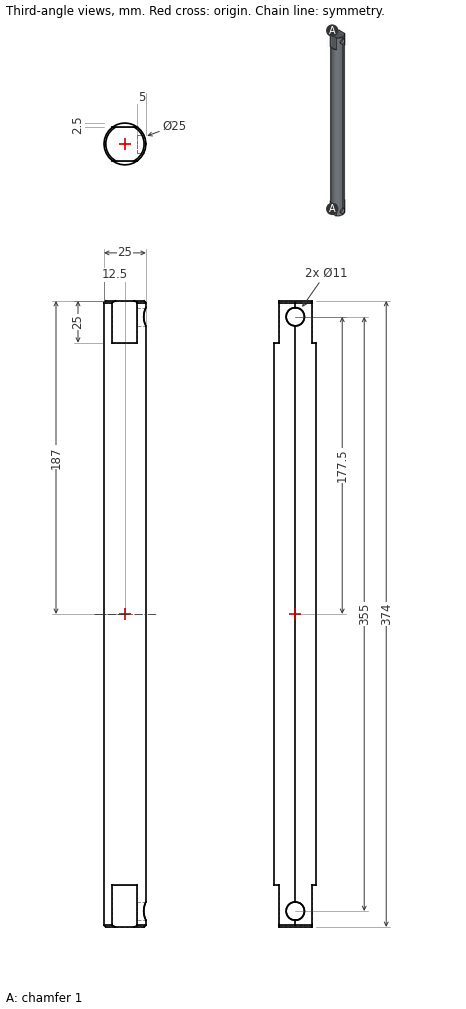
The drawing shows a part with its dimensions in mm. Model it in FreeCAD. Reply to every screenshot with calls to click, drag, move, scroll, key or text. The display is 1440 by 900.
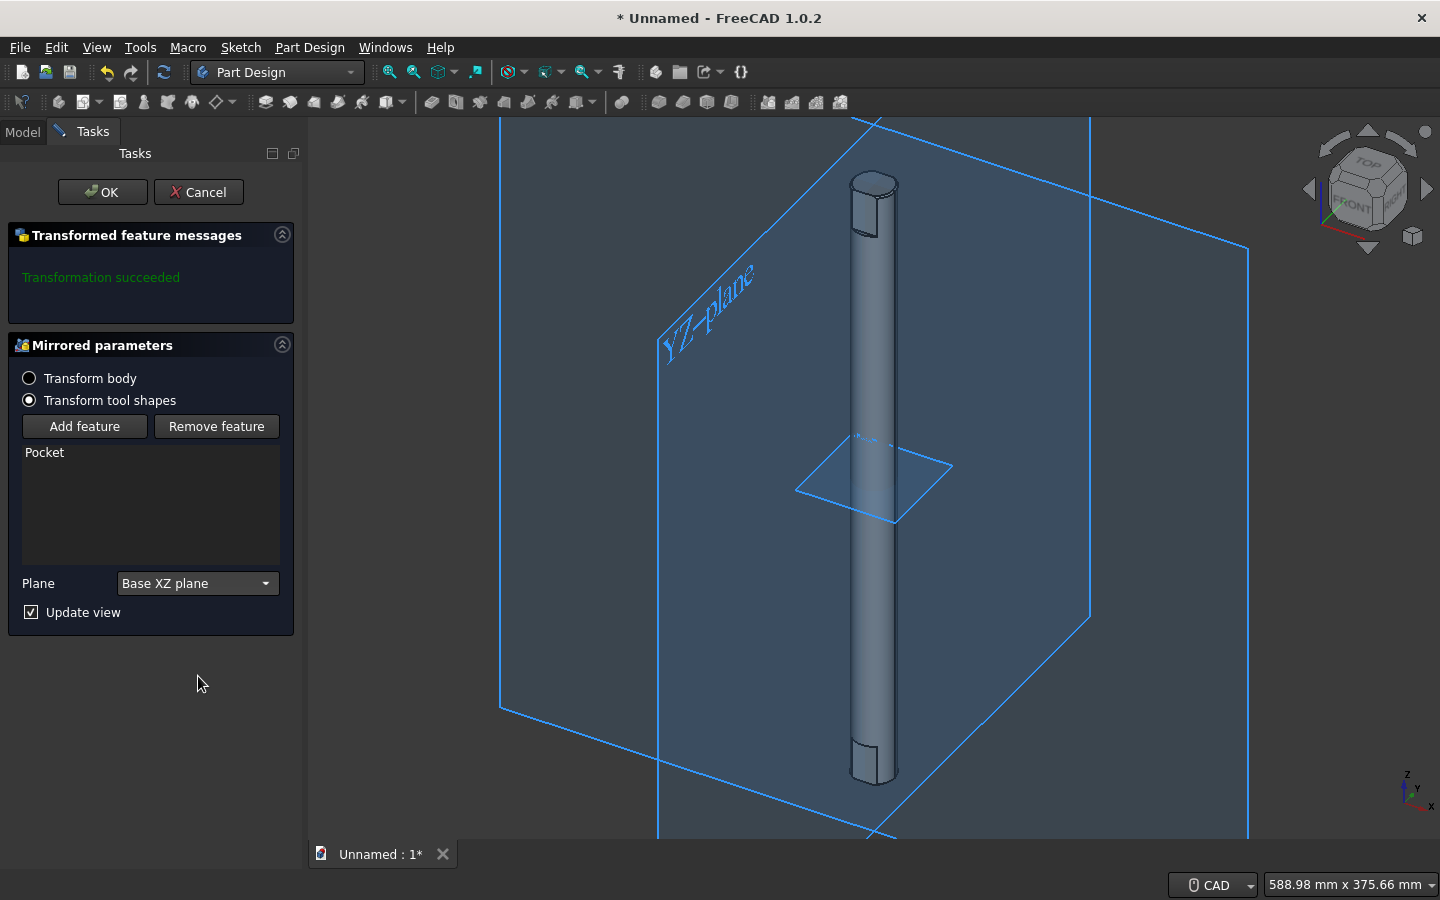
click(103, 192)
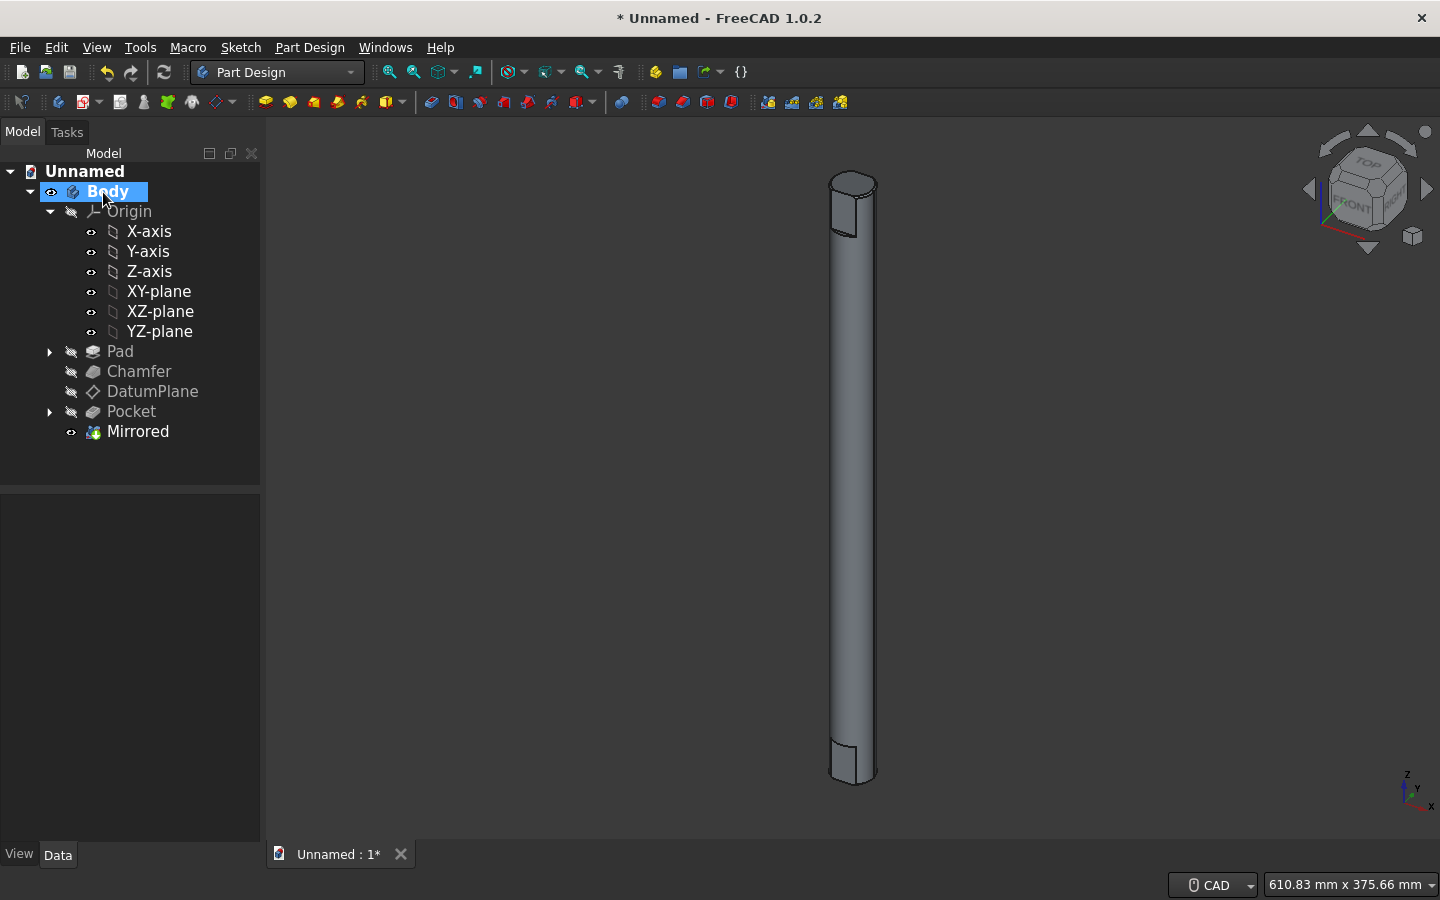
click(136, 332)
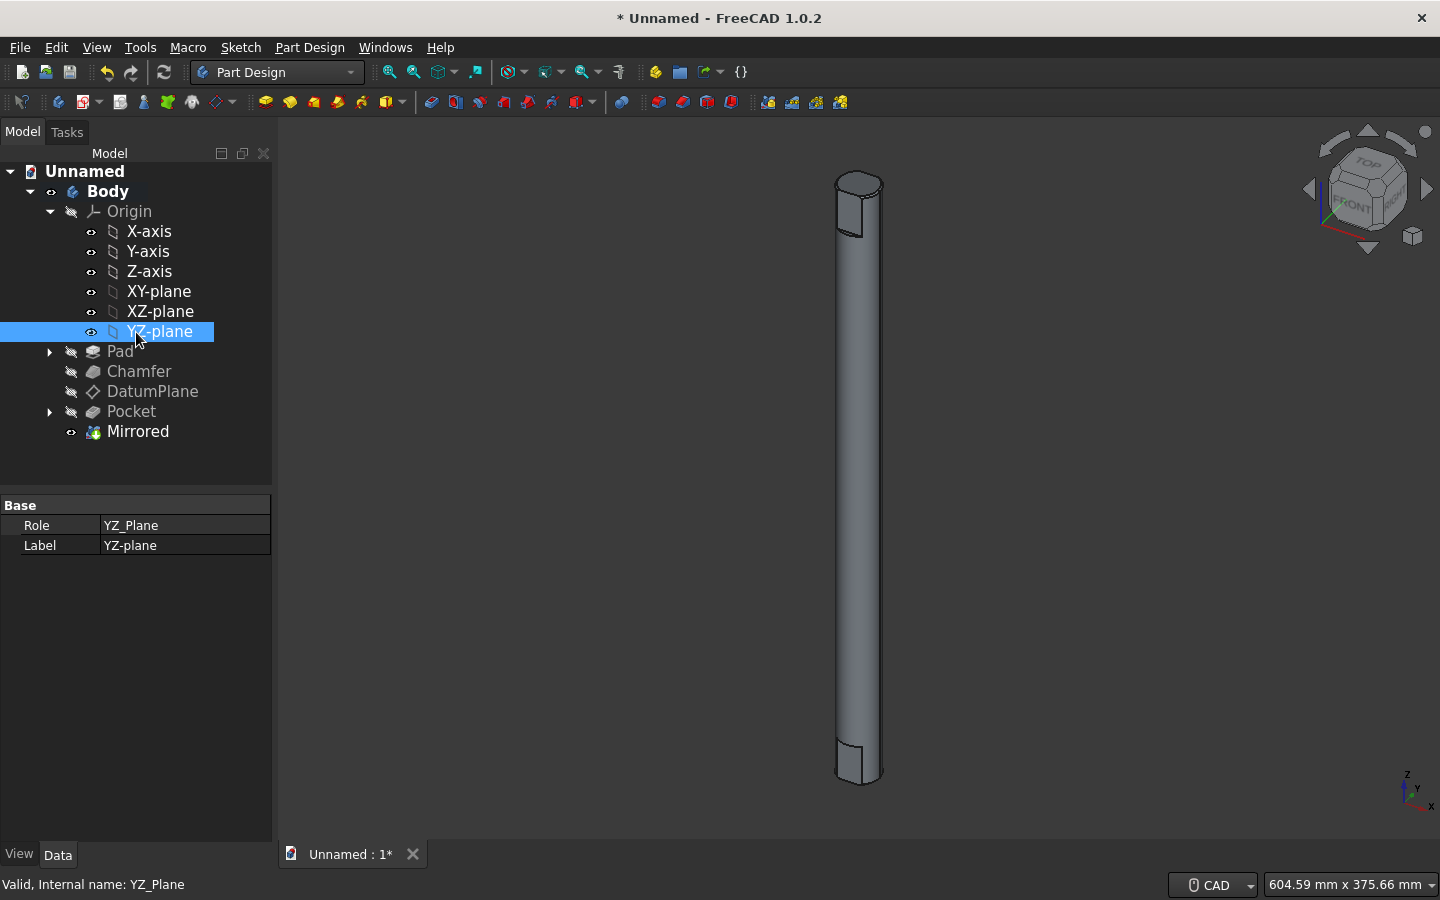
click(216, 102)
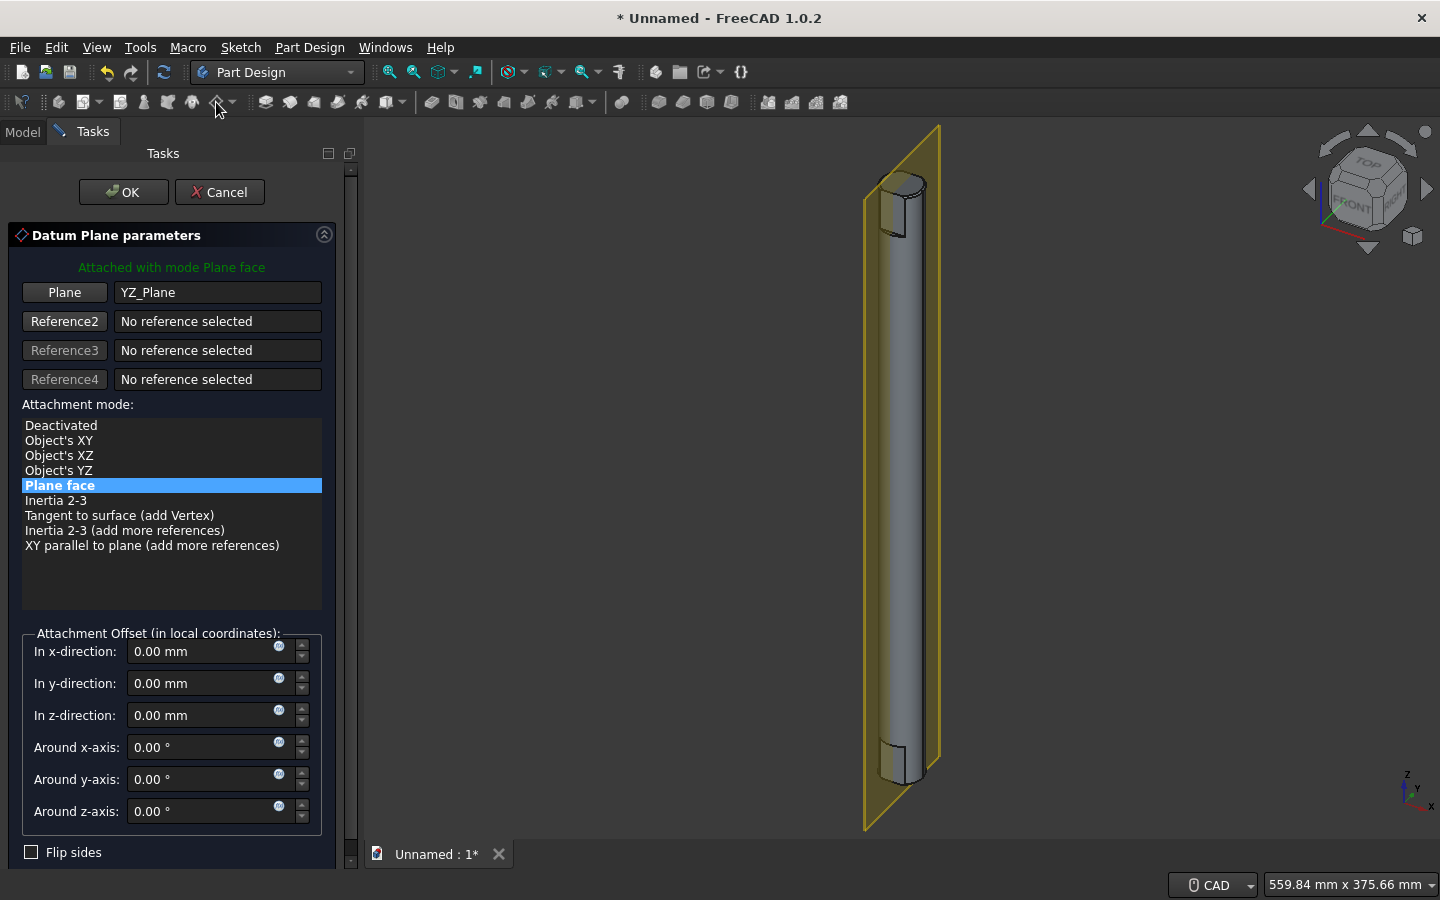
triple_click(210, 715)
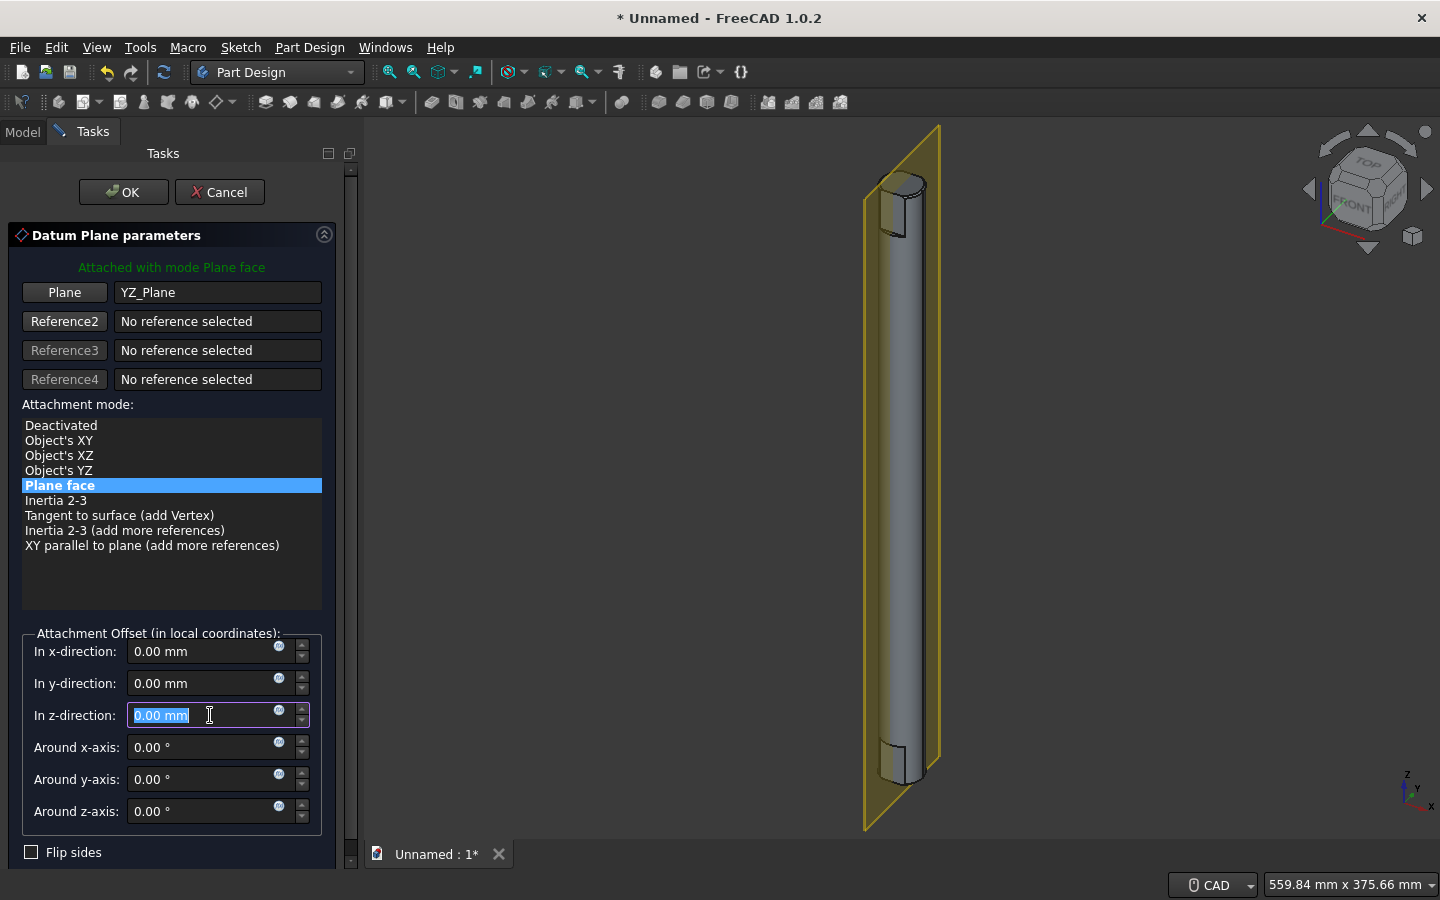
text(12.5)
key(Tab)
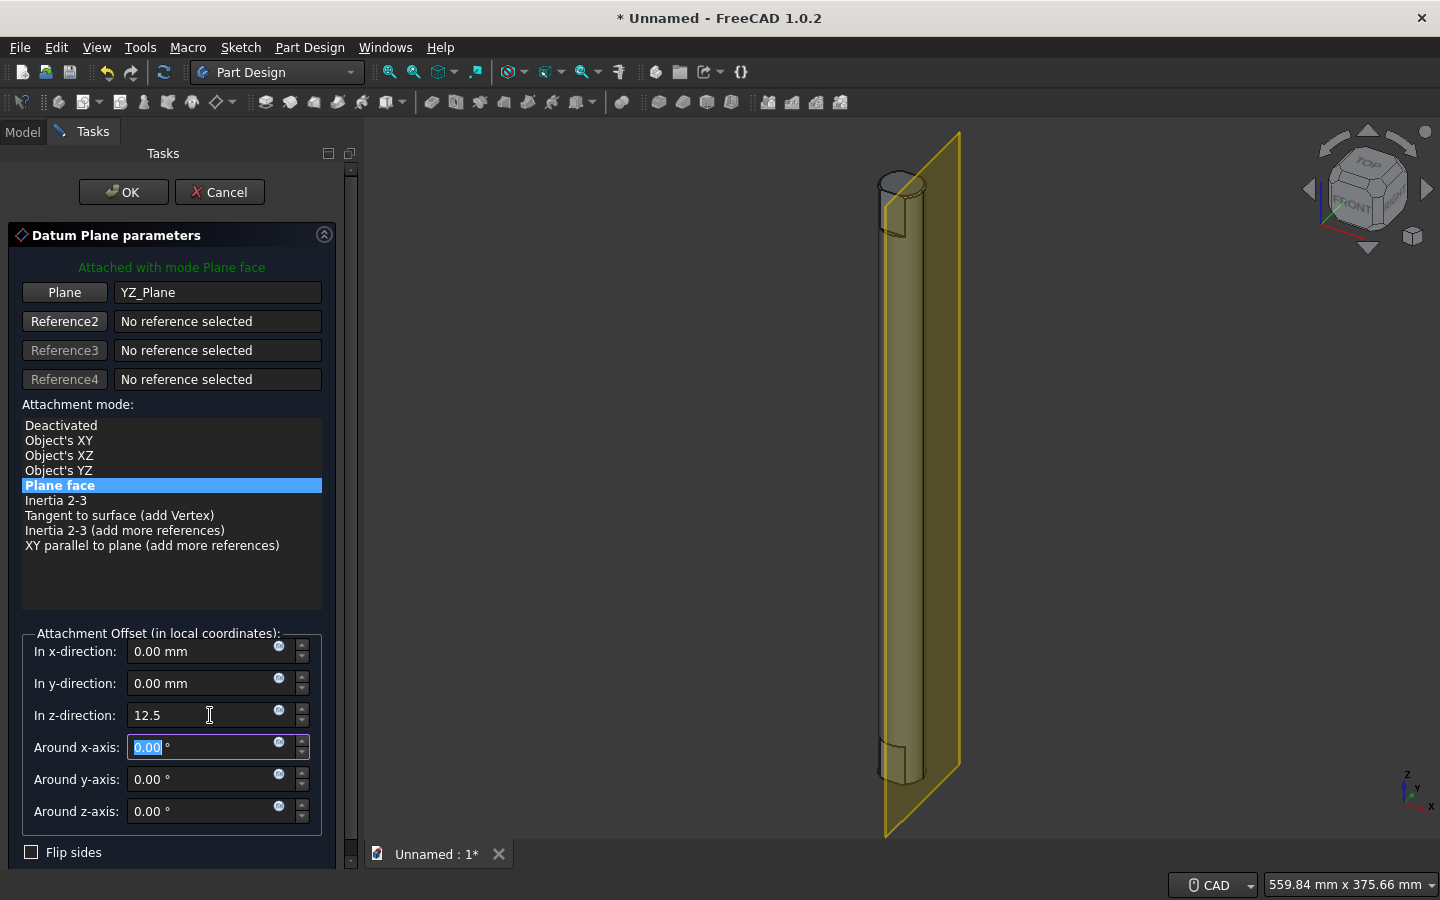
click(124, 192)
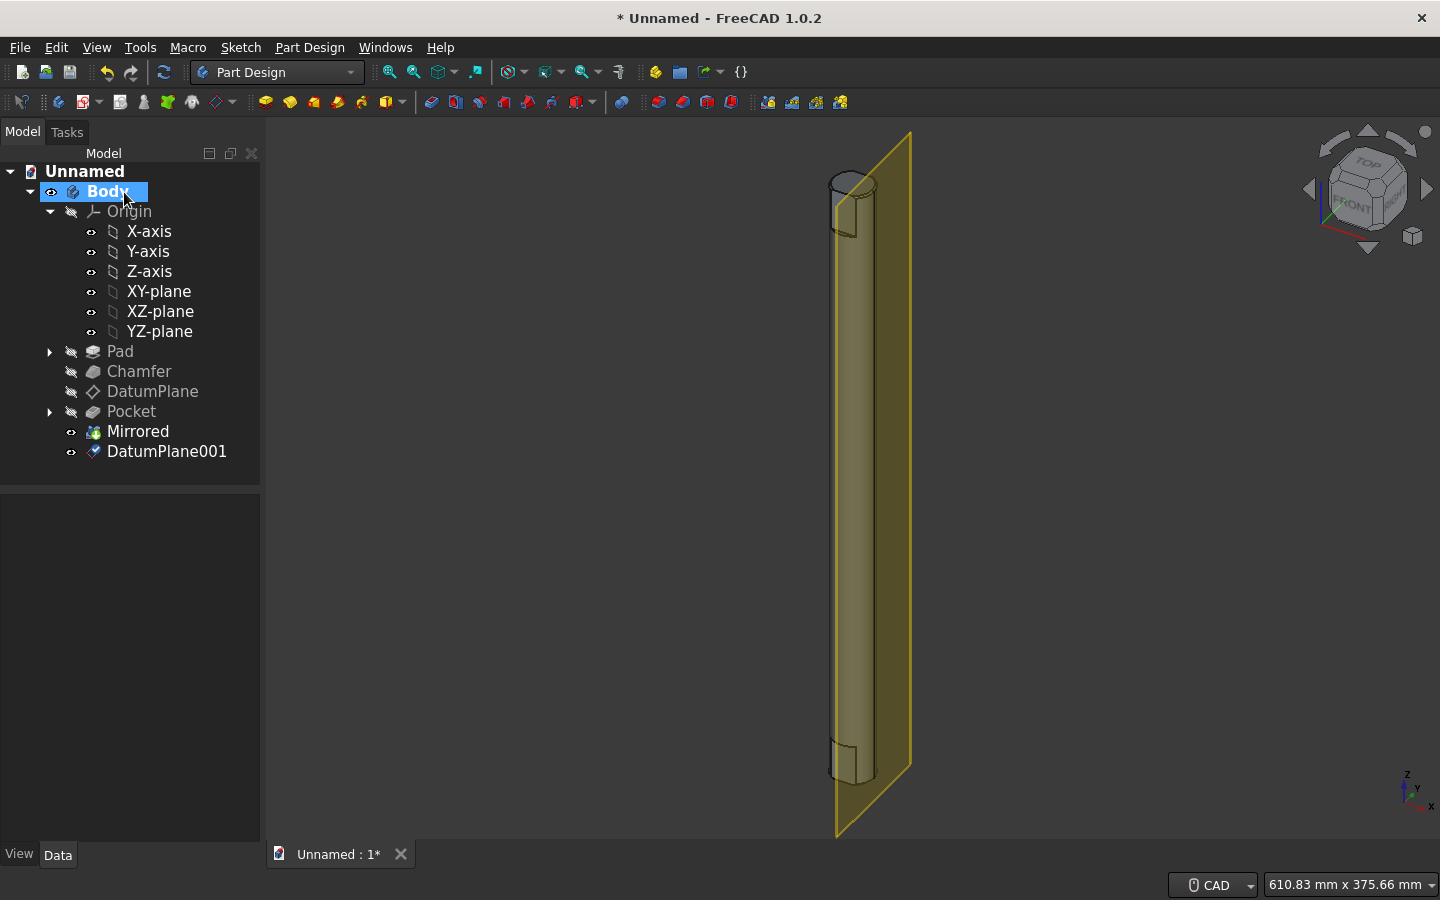
click(116, 452)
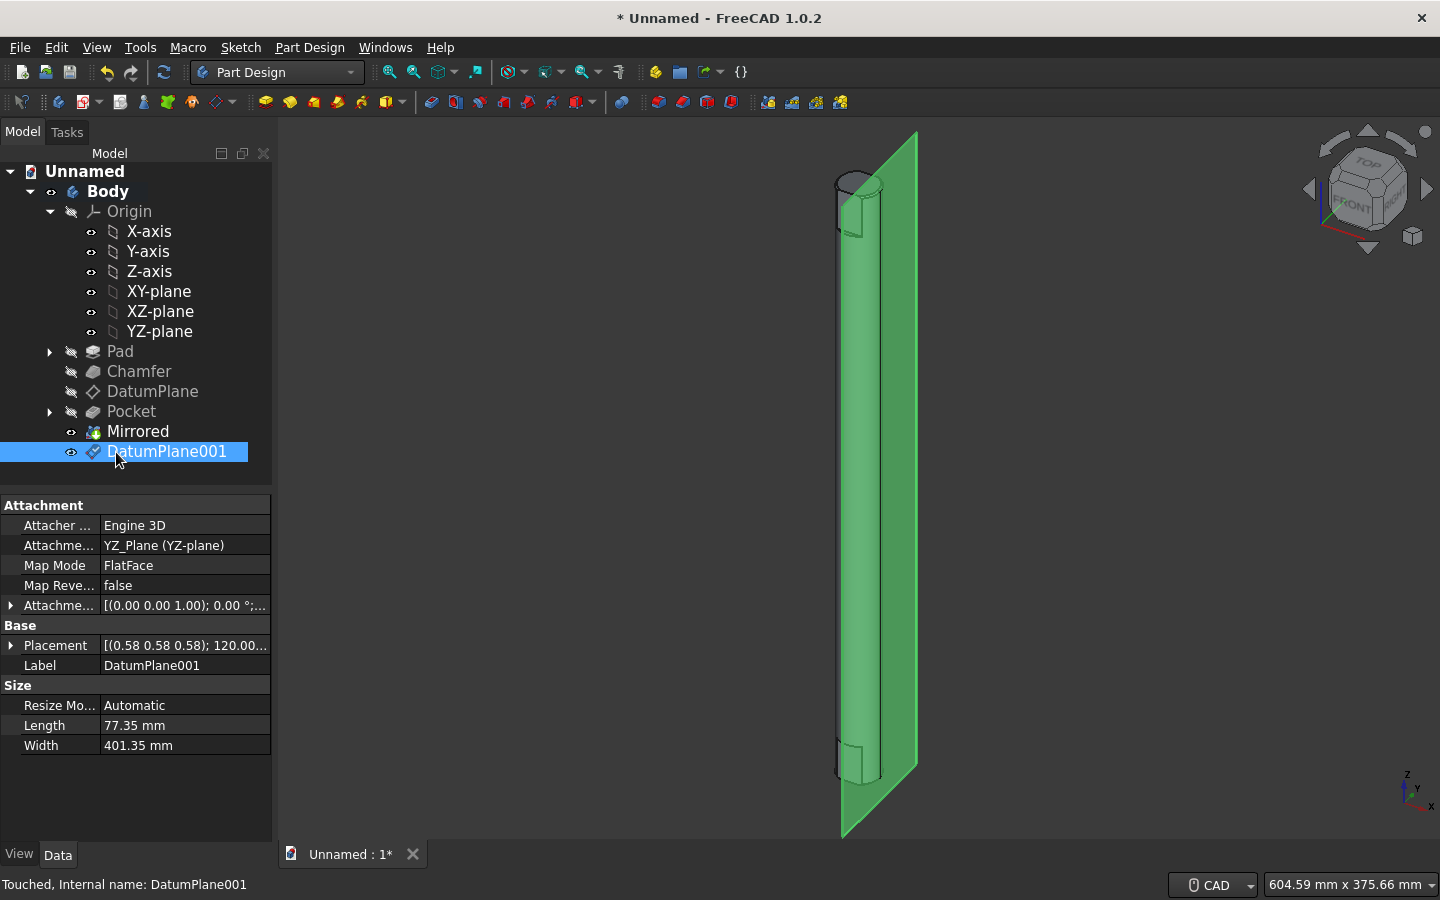
click(84, 102)